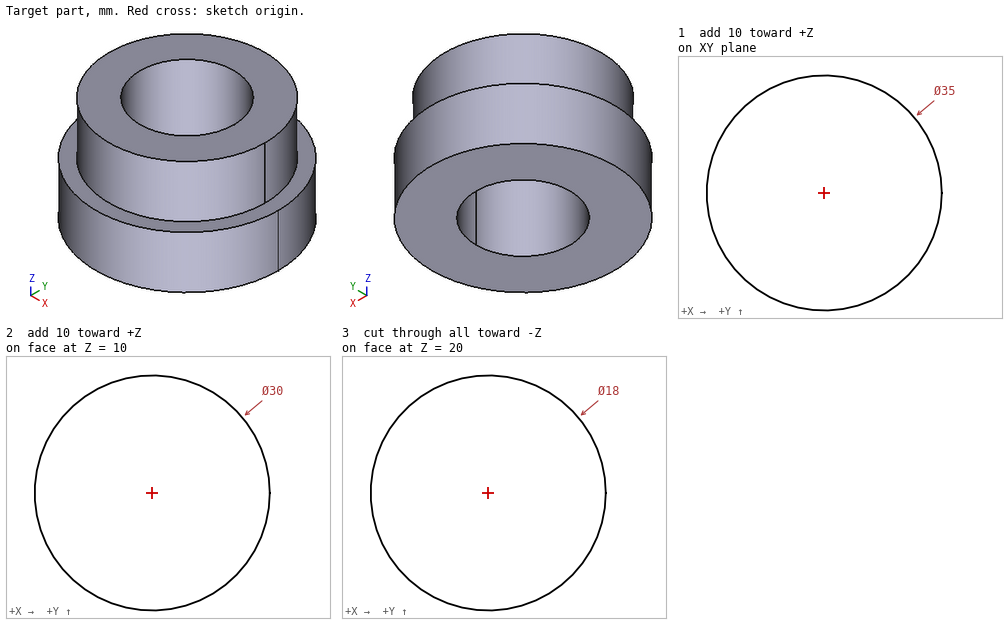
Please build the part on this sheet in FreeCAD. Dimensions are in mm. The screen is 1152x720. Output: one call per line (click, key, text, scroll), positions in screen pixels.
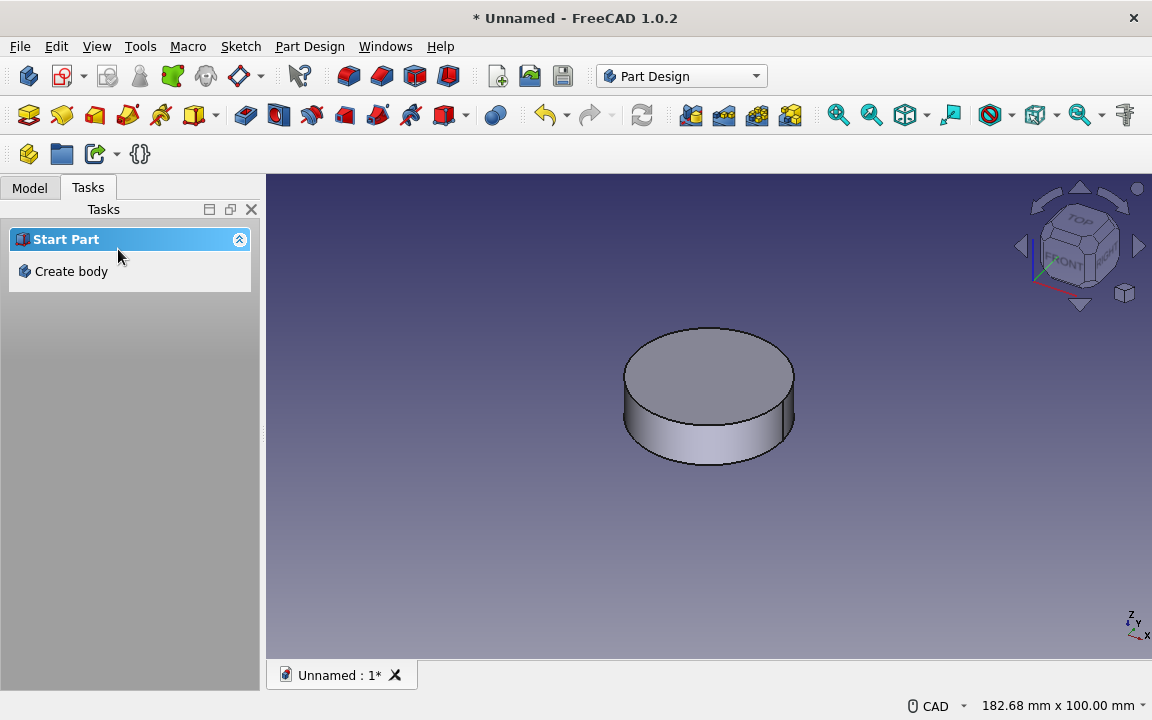
click(839, 116)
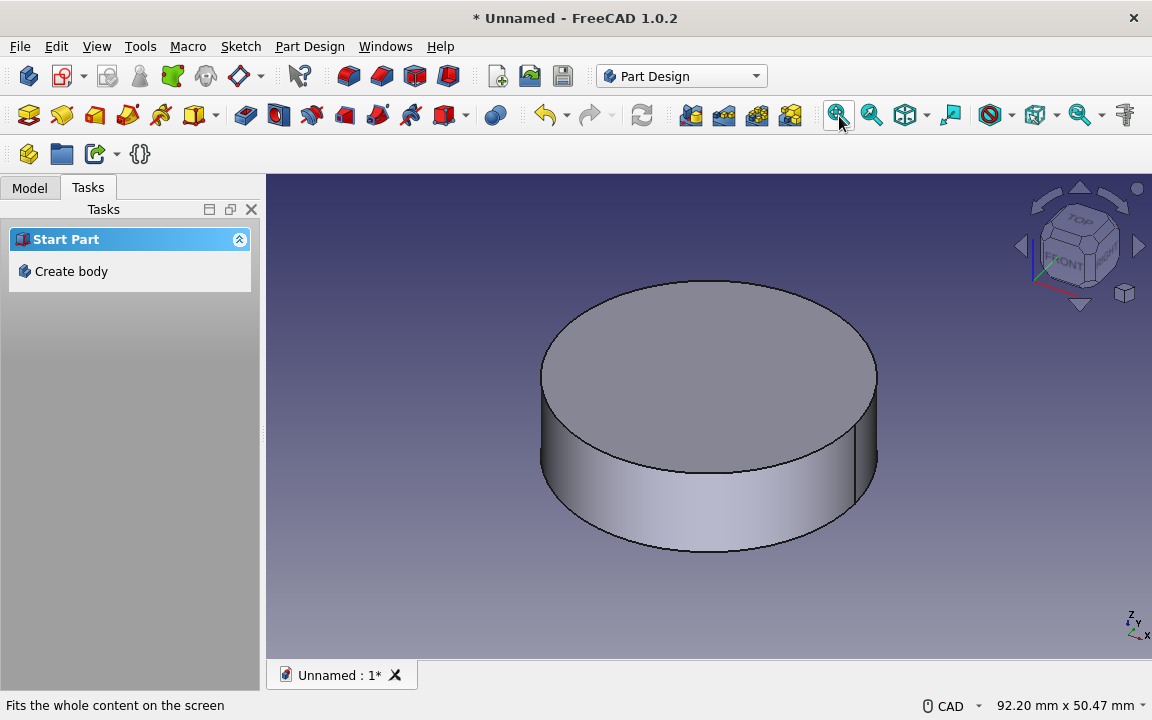
click(709, 376)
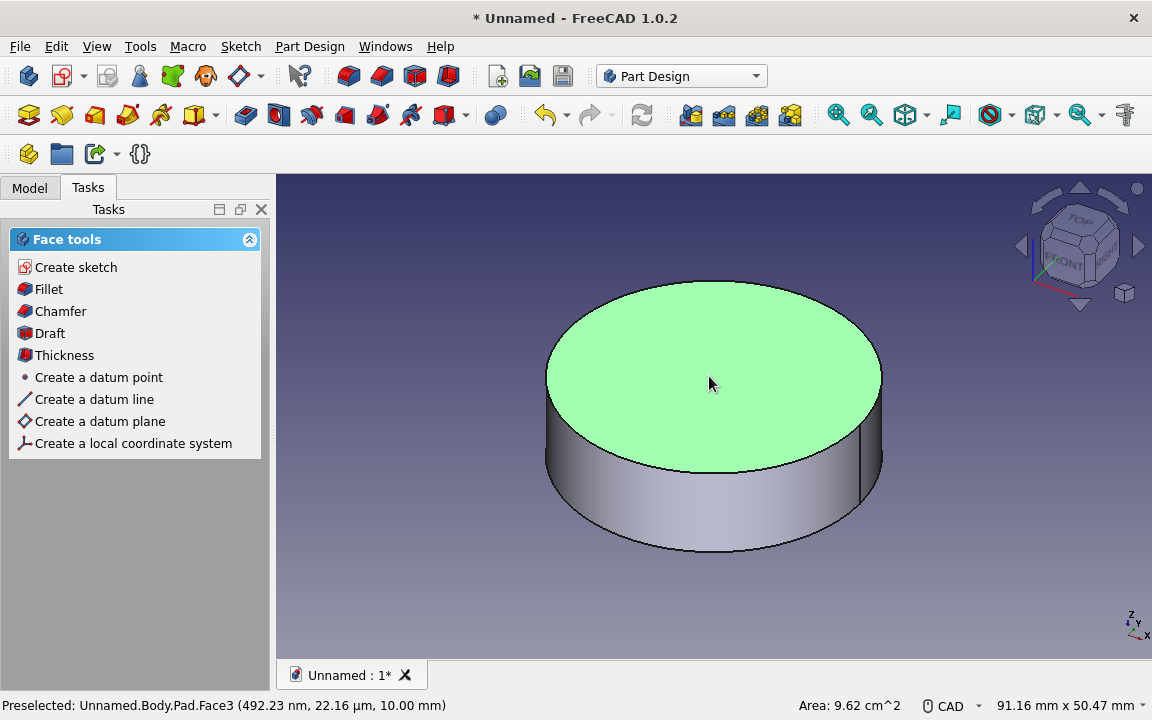
click(62, 76)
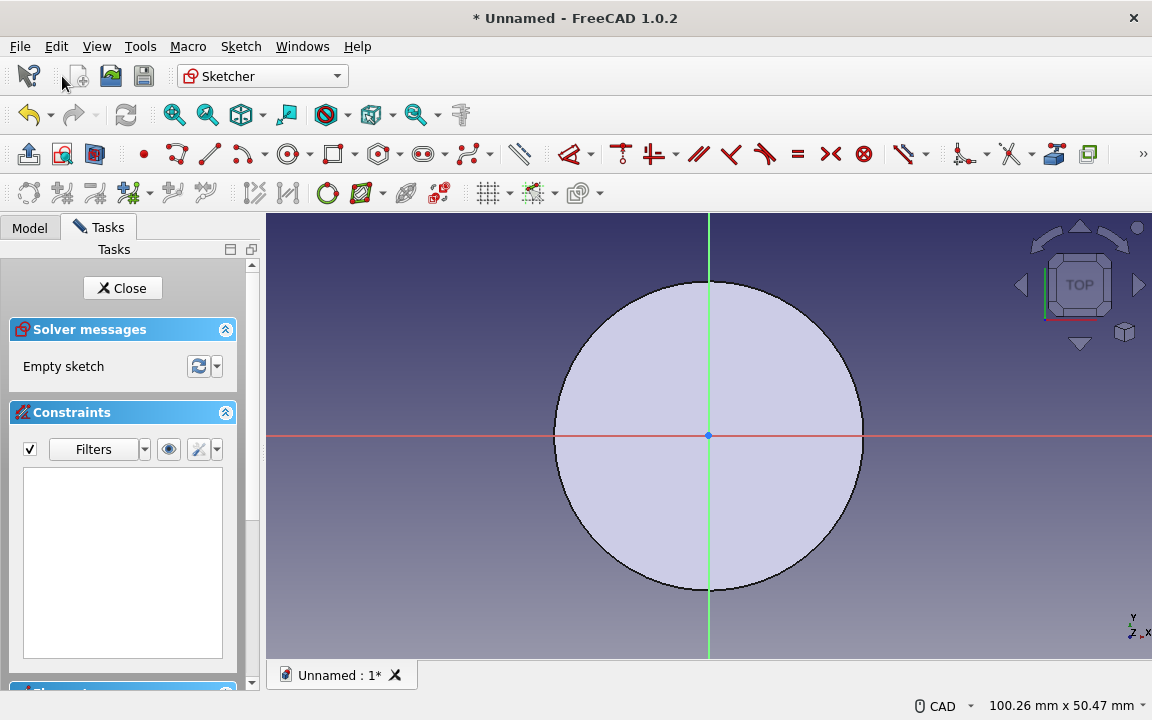
click(288, 154)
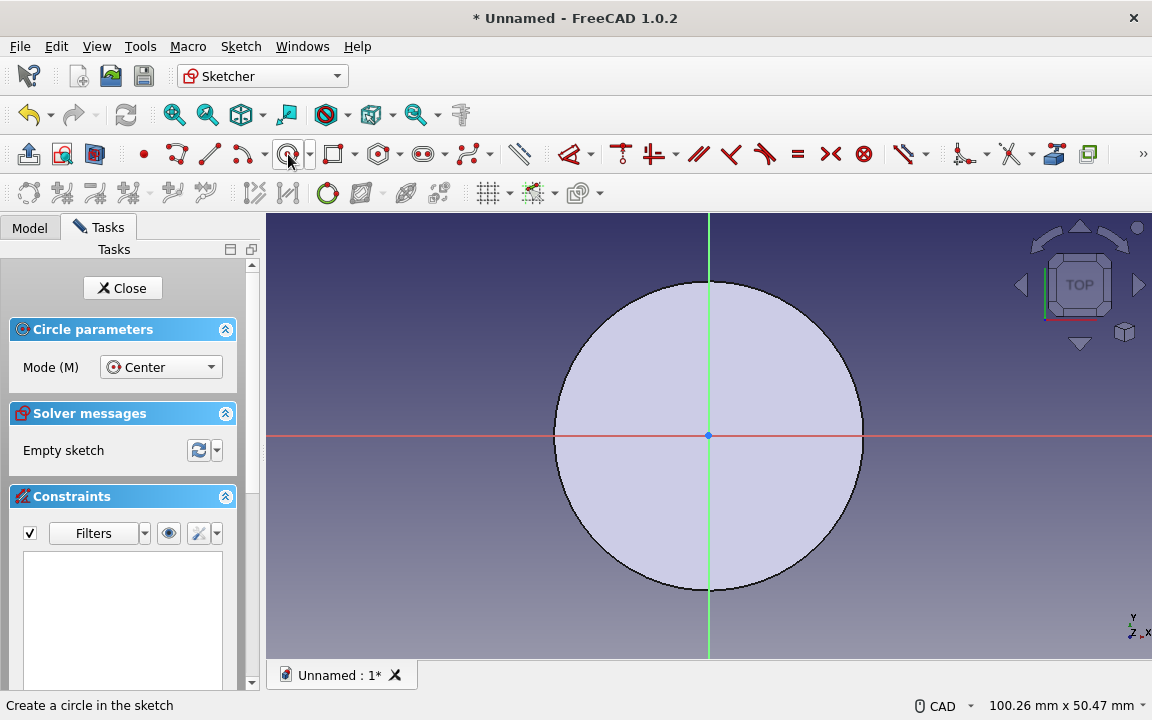
click(709, 436)
move(803, 342)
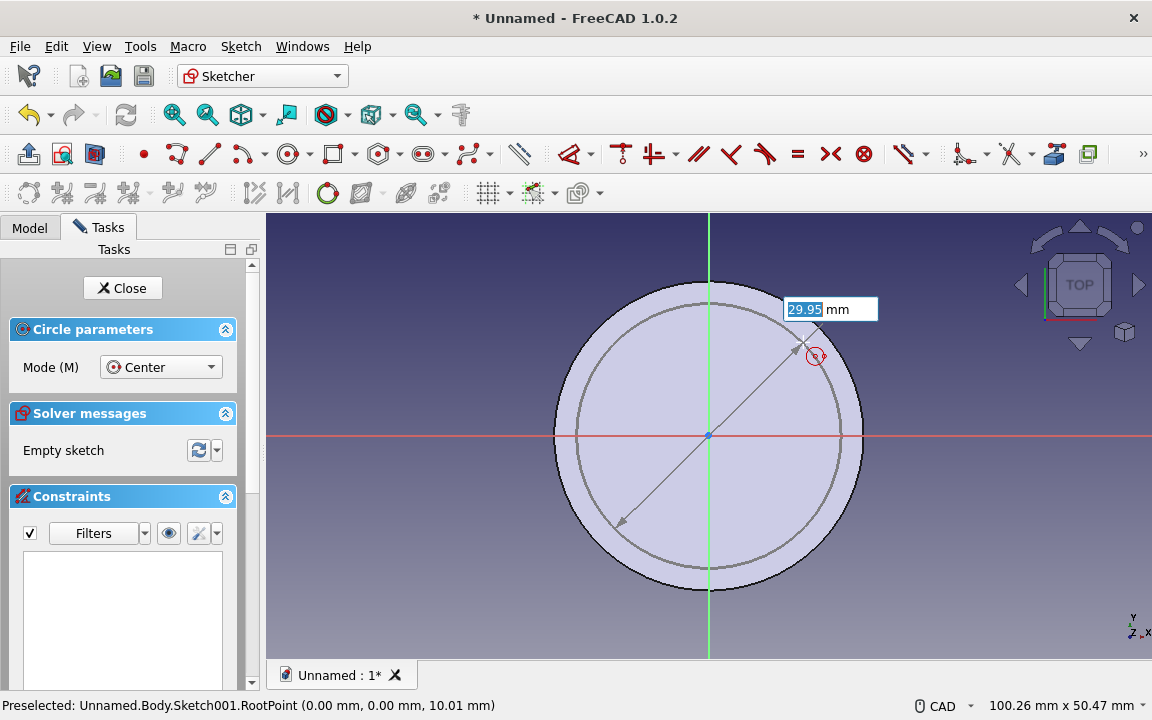
text(30)
key(Return)
key(Escape)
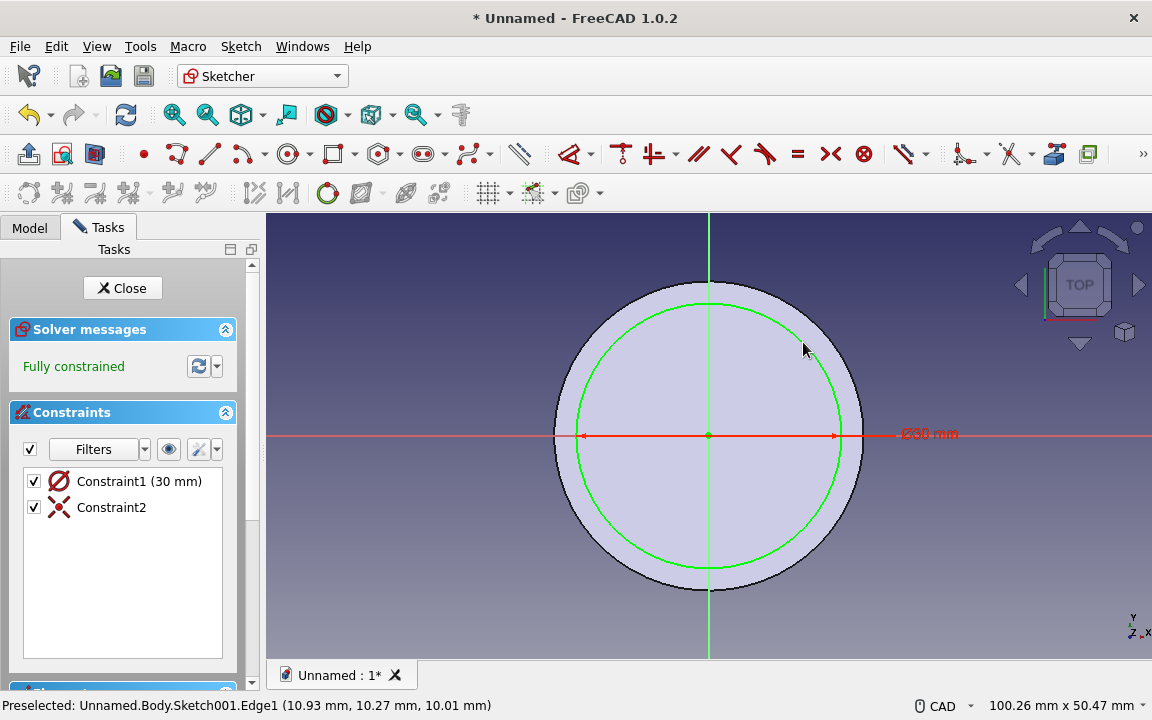
click(123, 288)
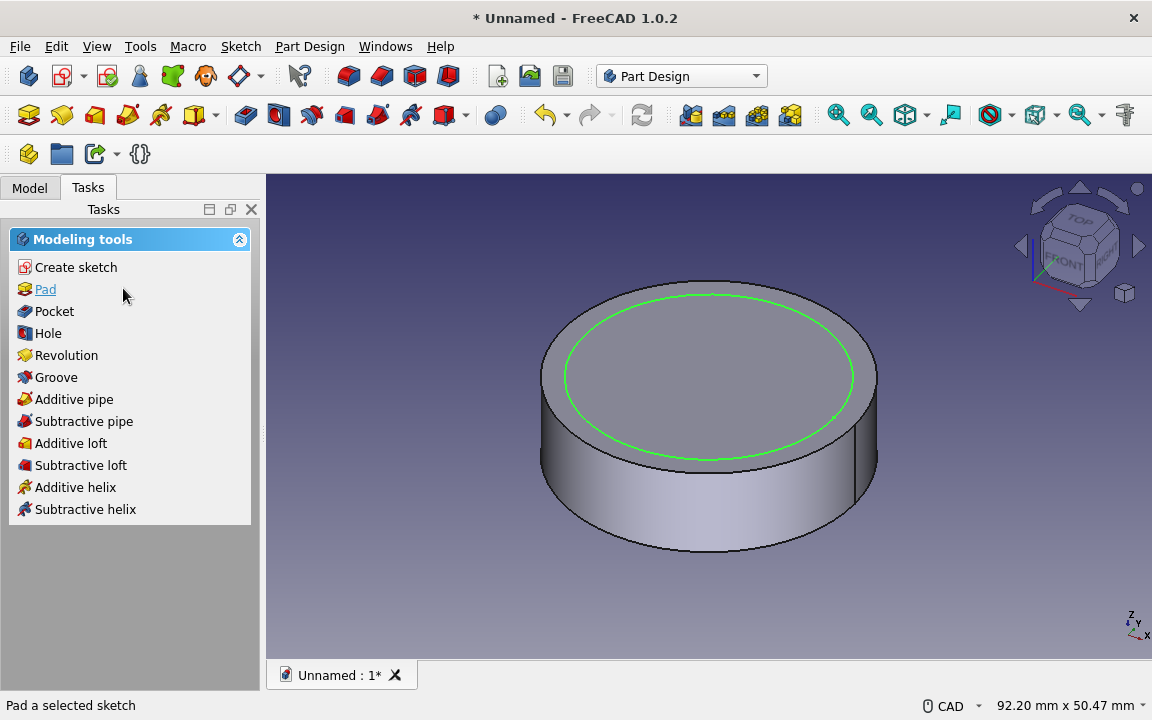
click(29, 116)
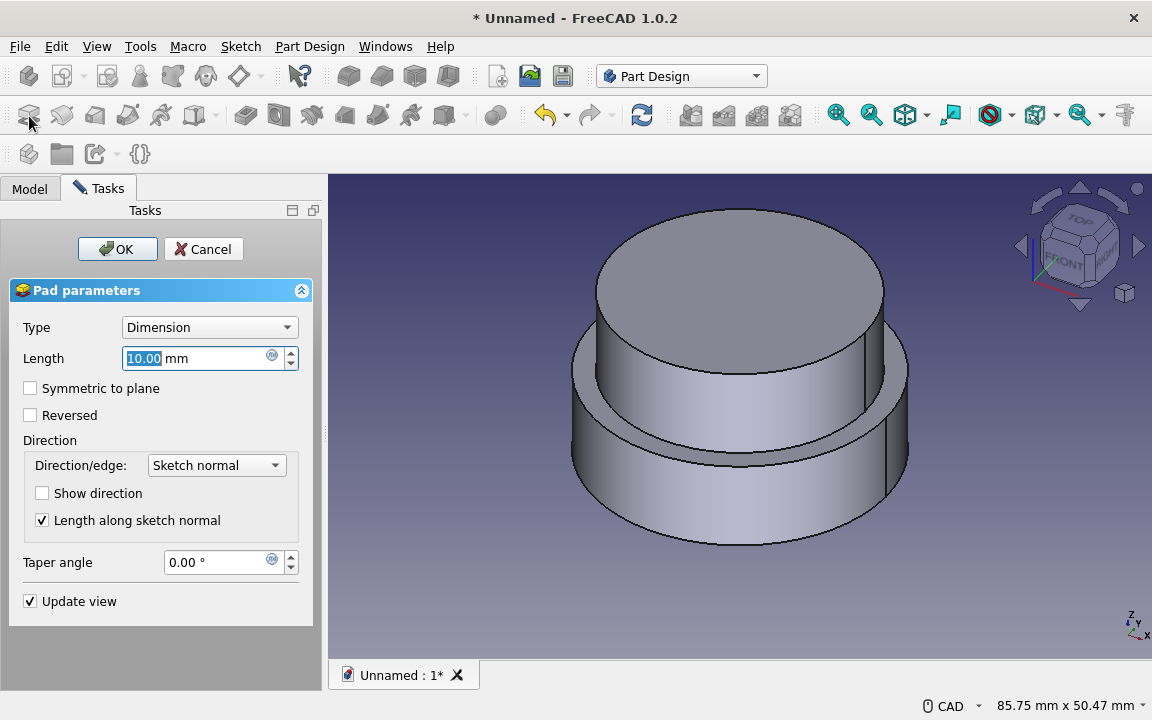
text(10)
key(Tab)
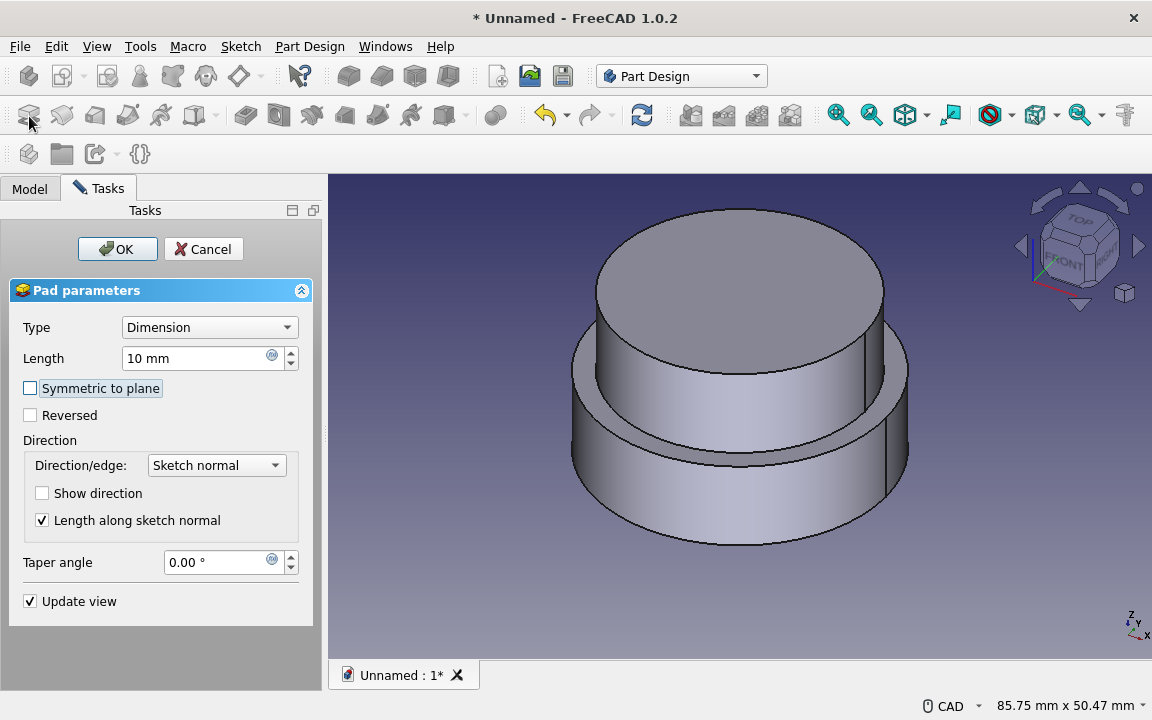
click(118, 249)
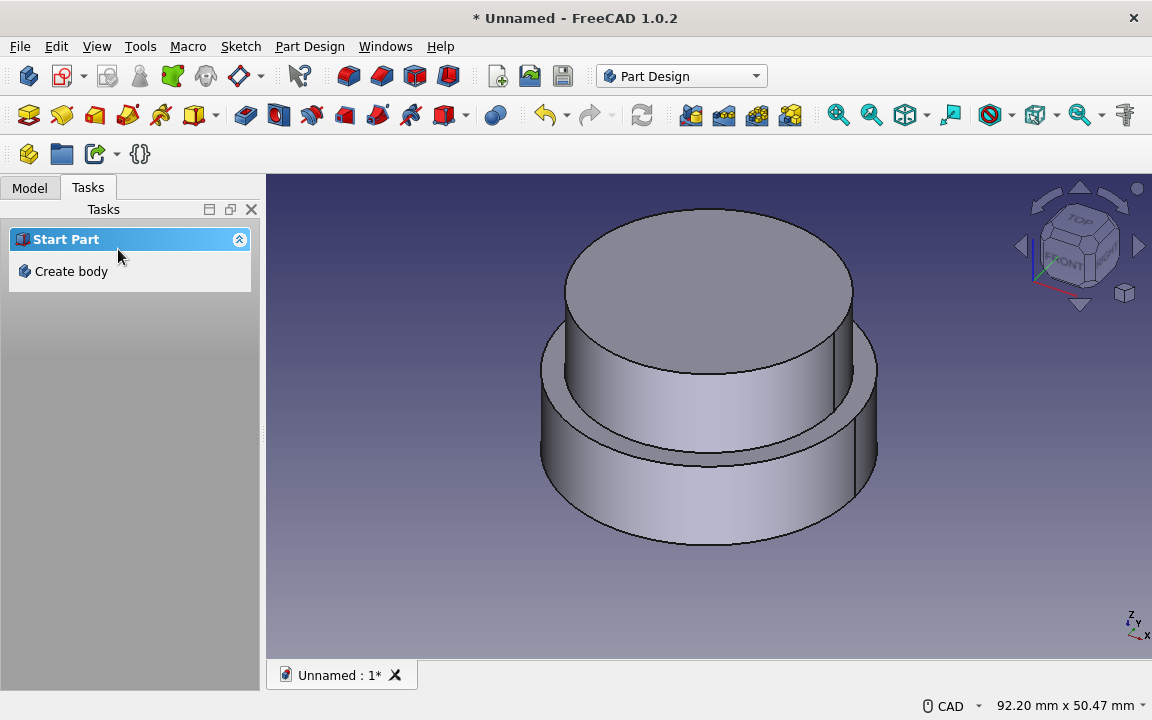
click(839, 116)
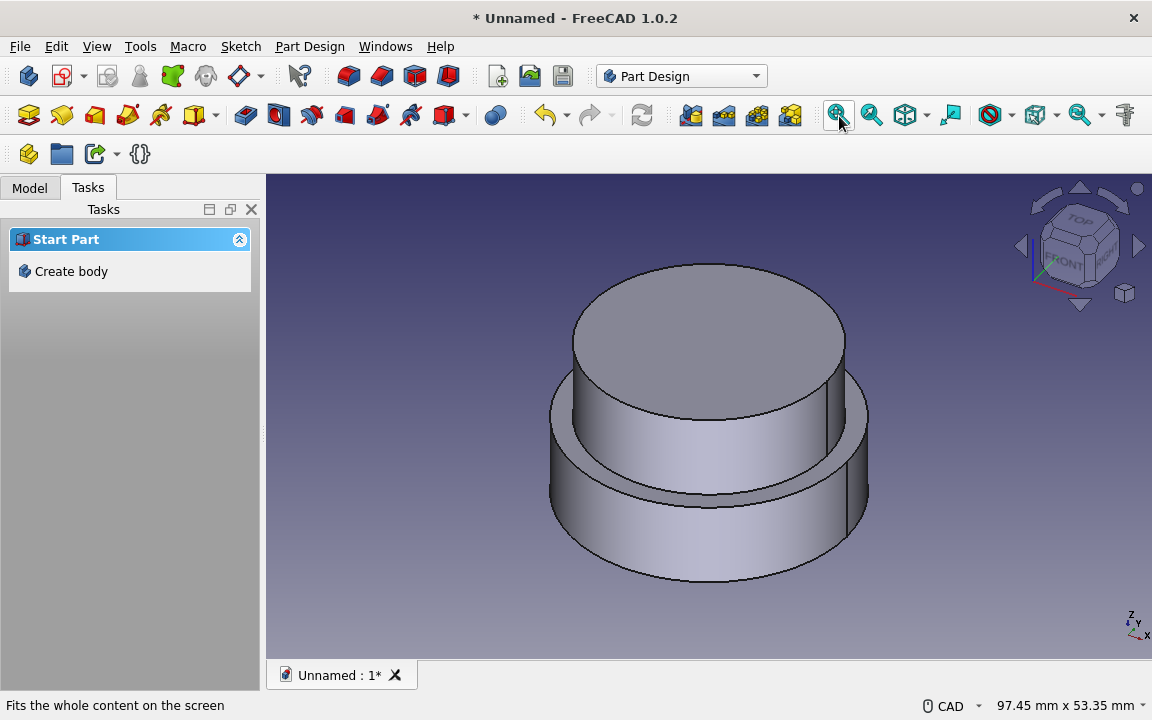
click(709, 341)